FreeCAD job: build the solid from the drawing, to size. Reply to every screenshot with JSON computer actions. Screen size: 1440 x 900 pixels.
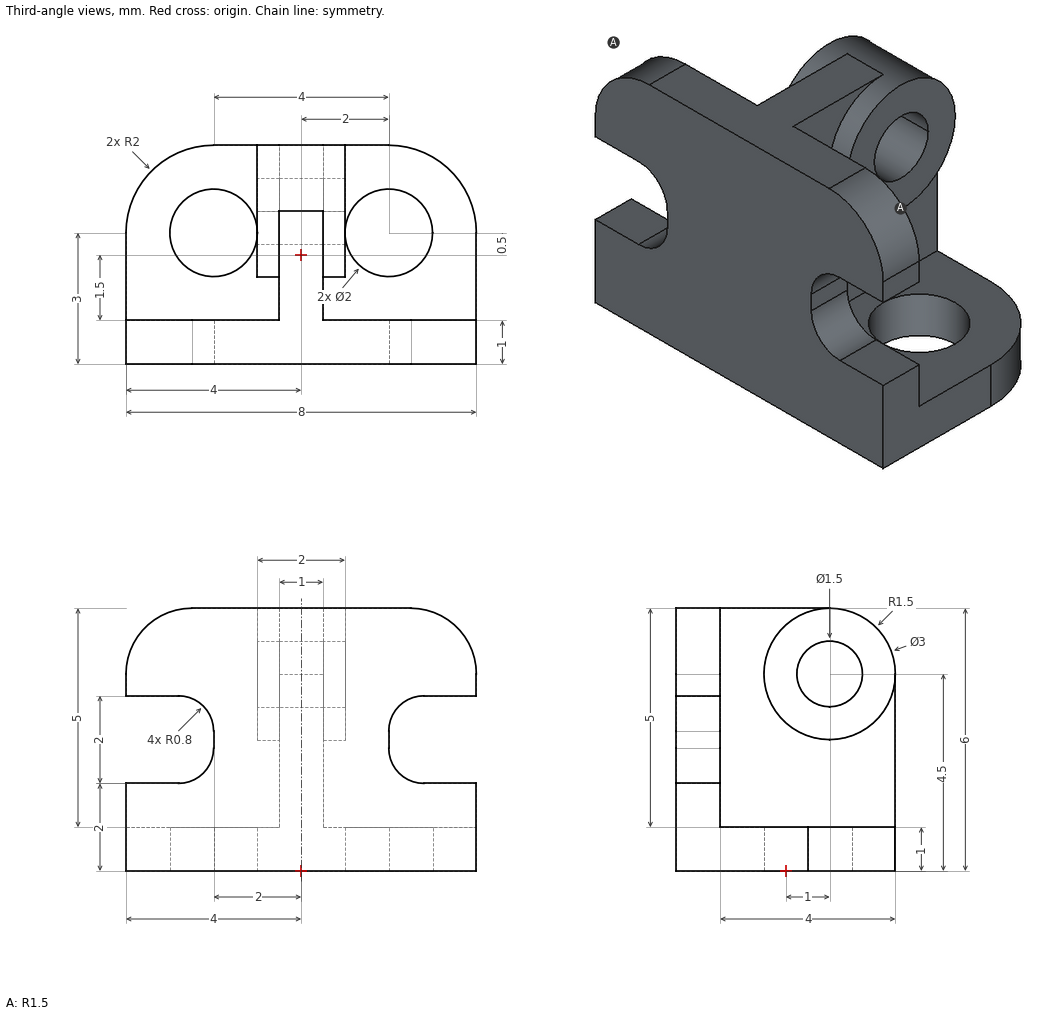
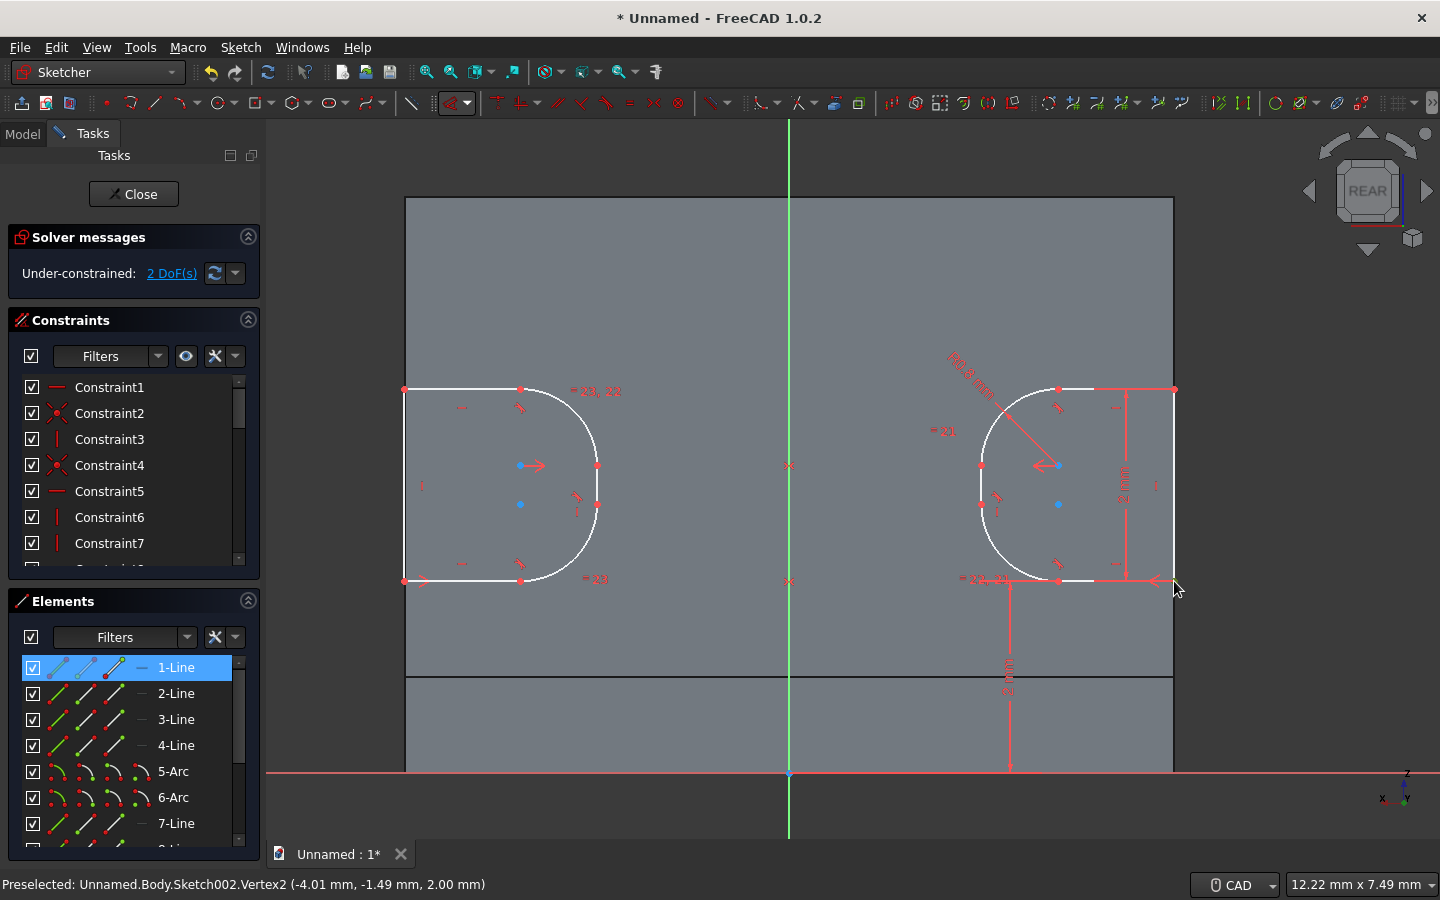
{"action": "left_click", "coordinate": [470, 104]}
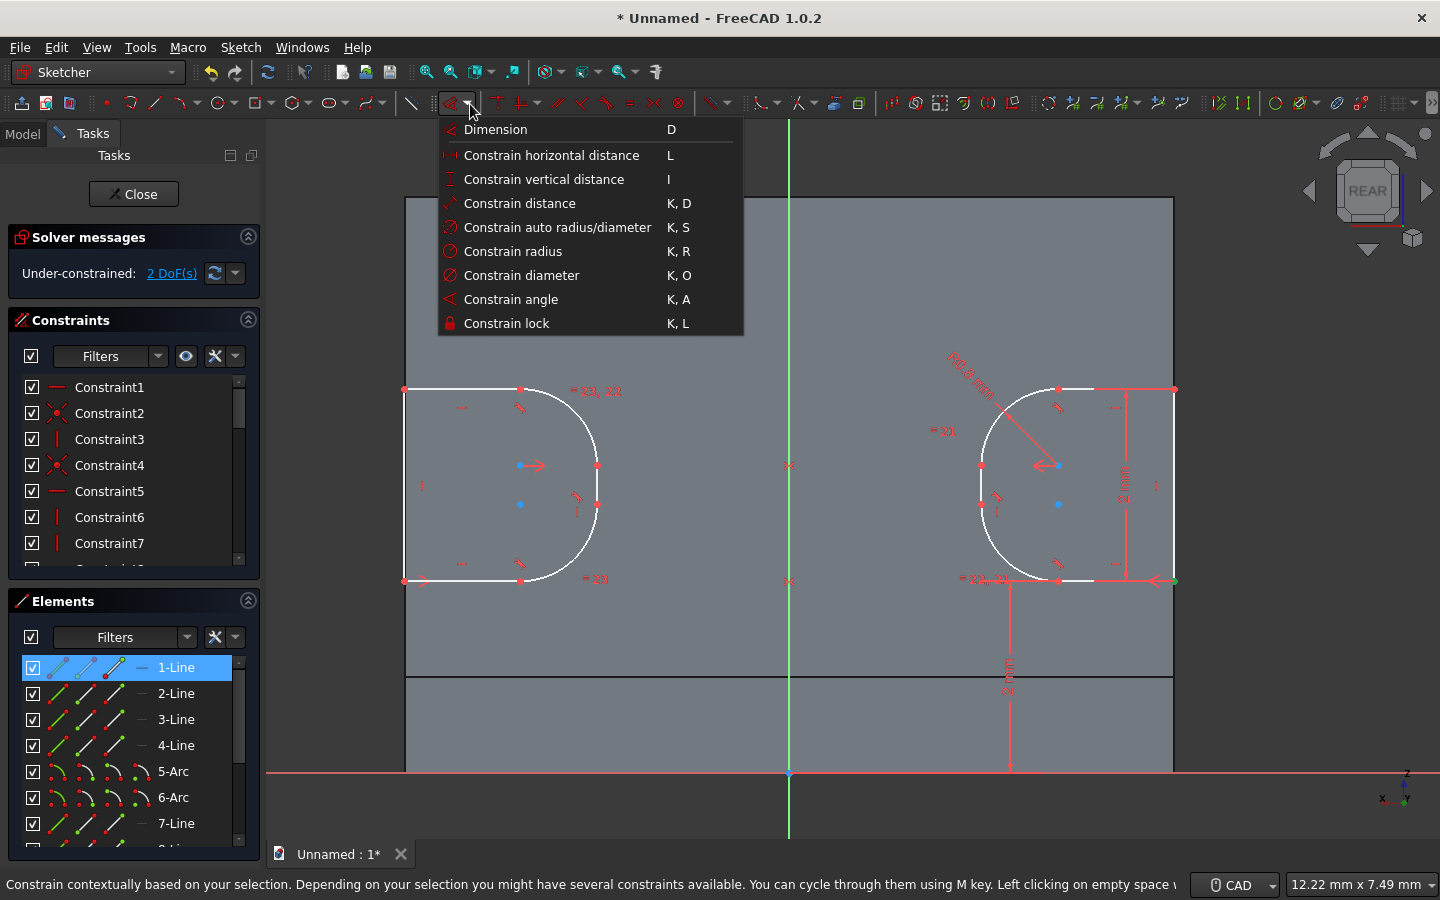
{"action": "left_click", "coordinate": [591, 155]}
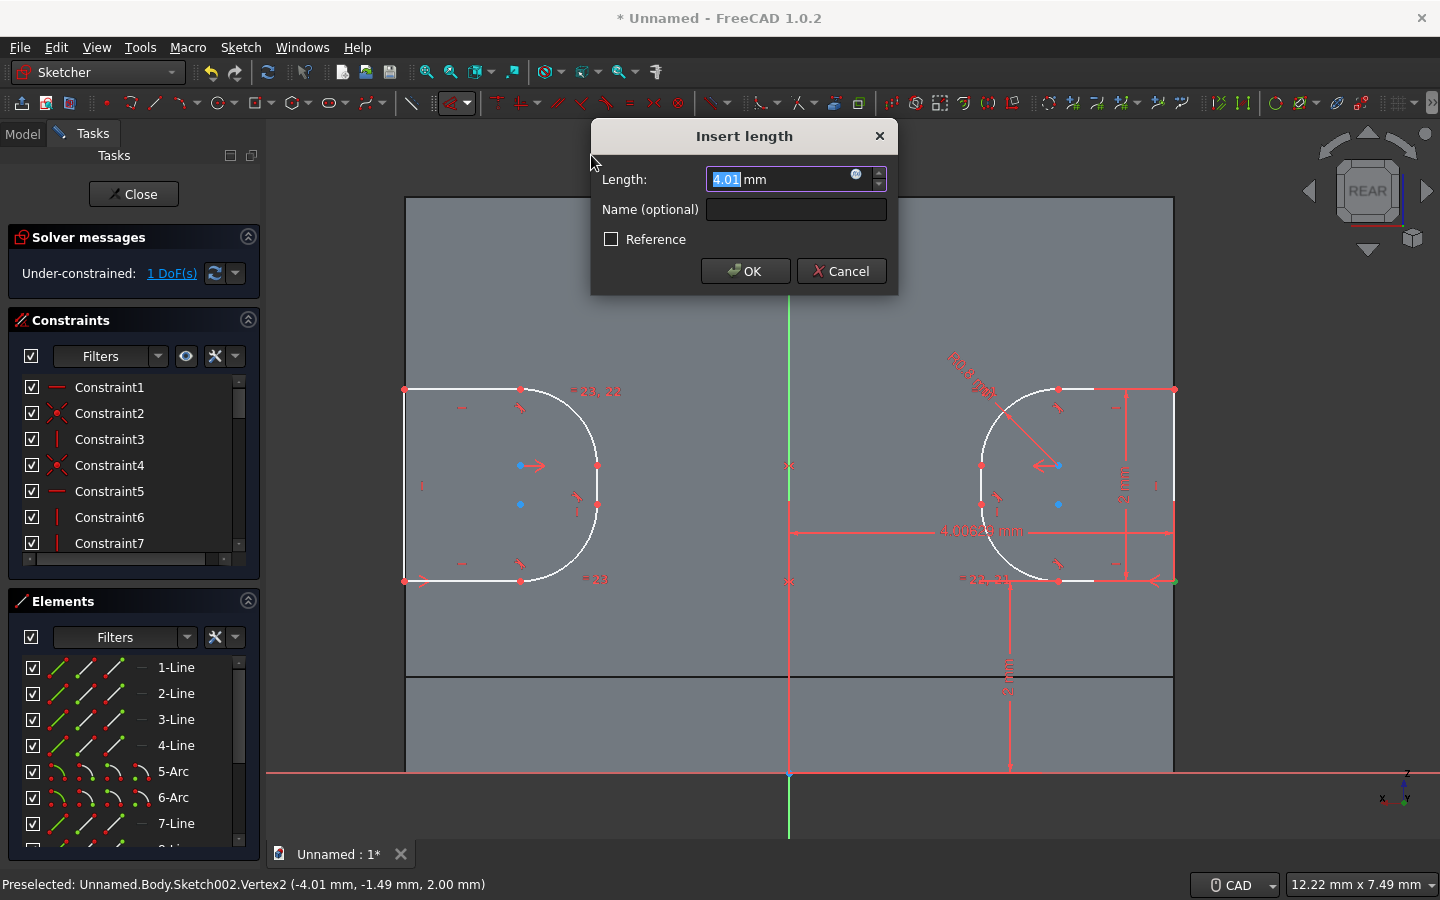
{"action": "type", "text": "4"}
{"action": "key", "text": "Return"}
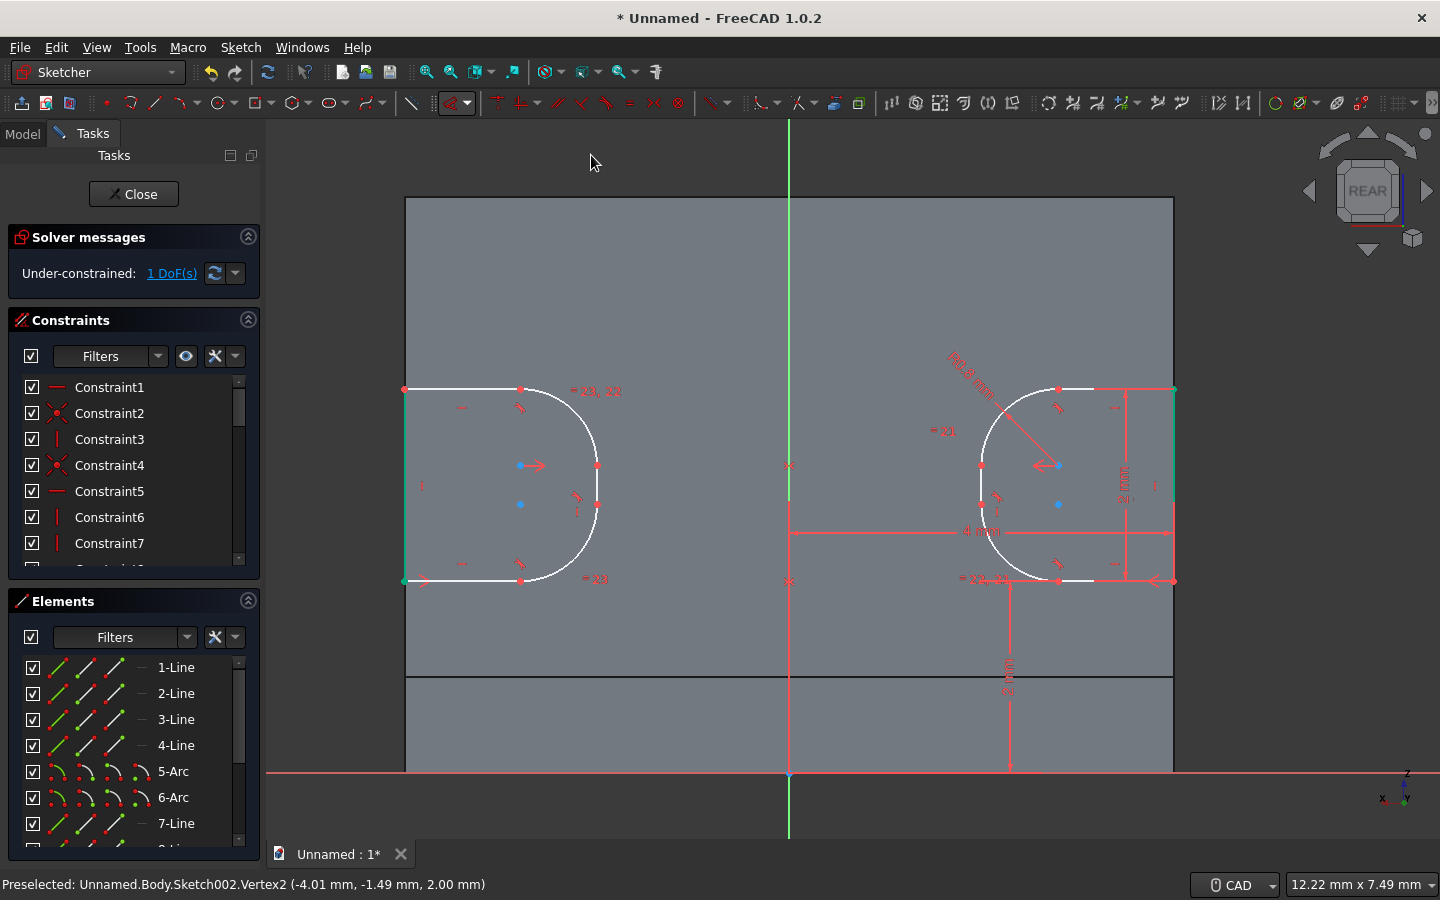
{"action": "left_click", "coordinate": [981, 466]}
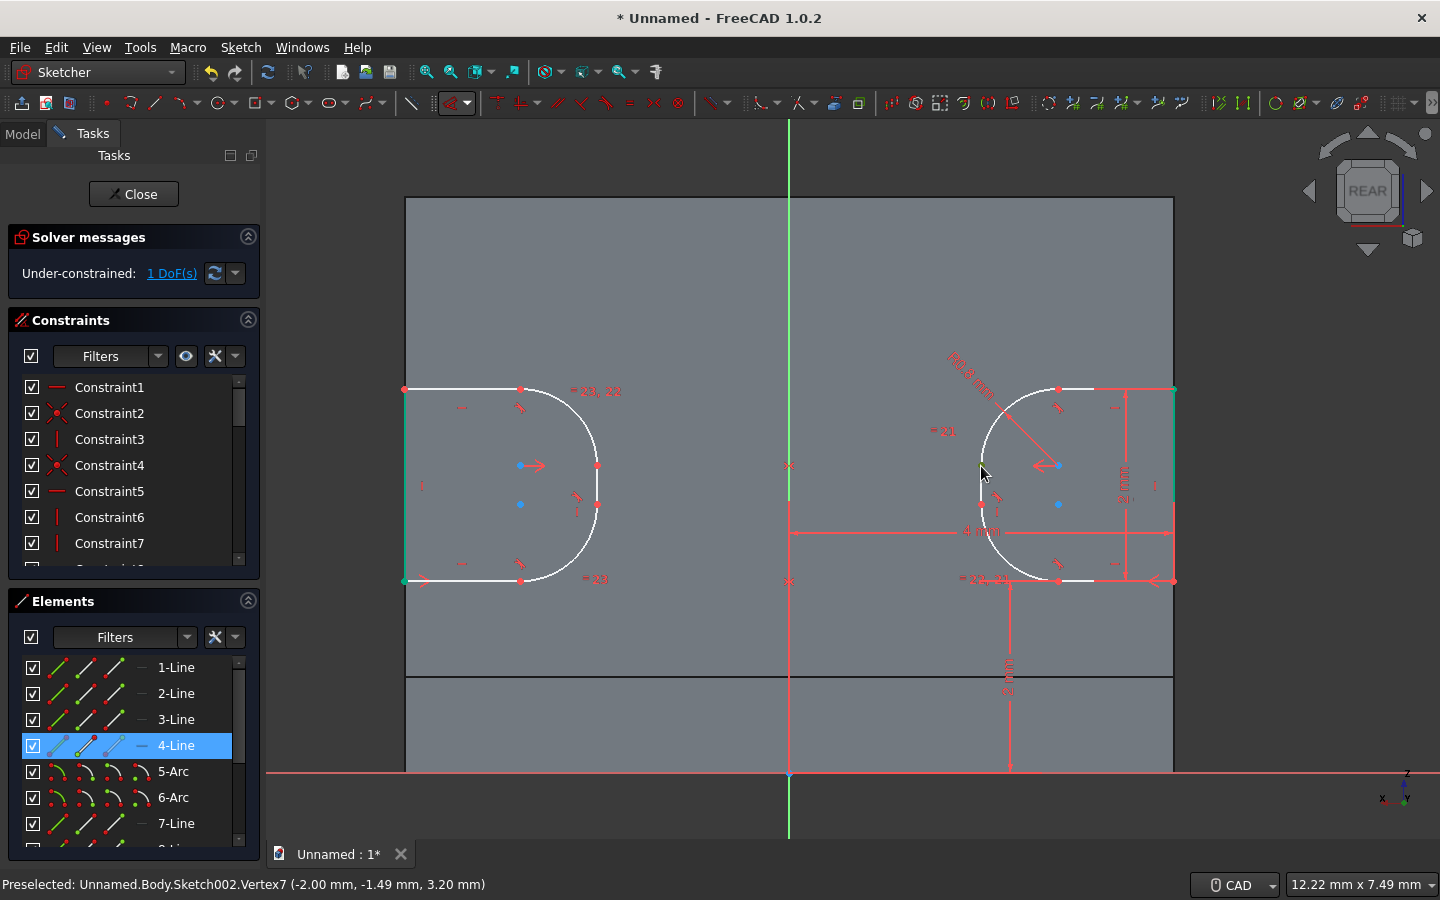
{"action": "left_click", "coordinate": [470, 104]}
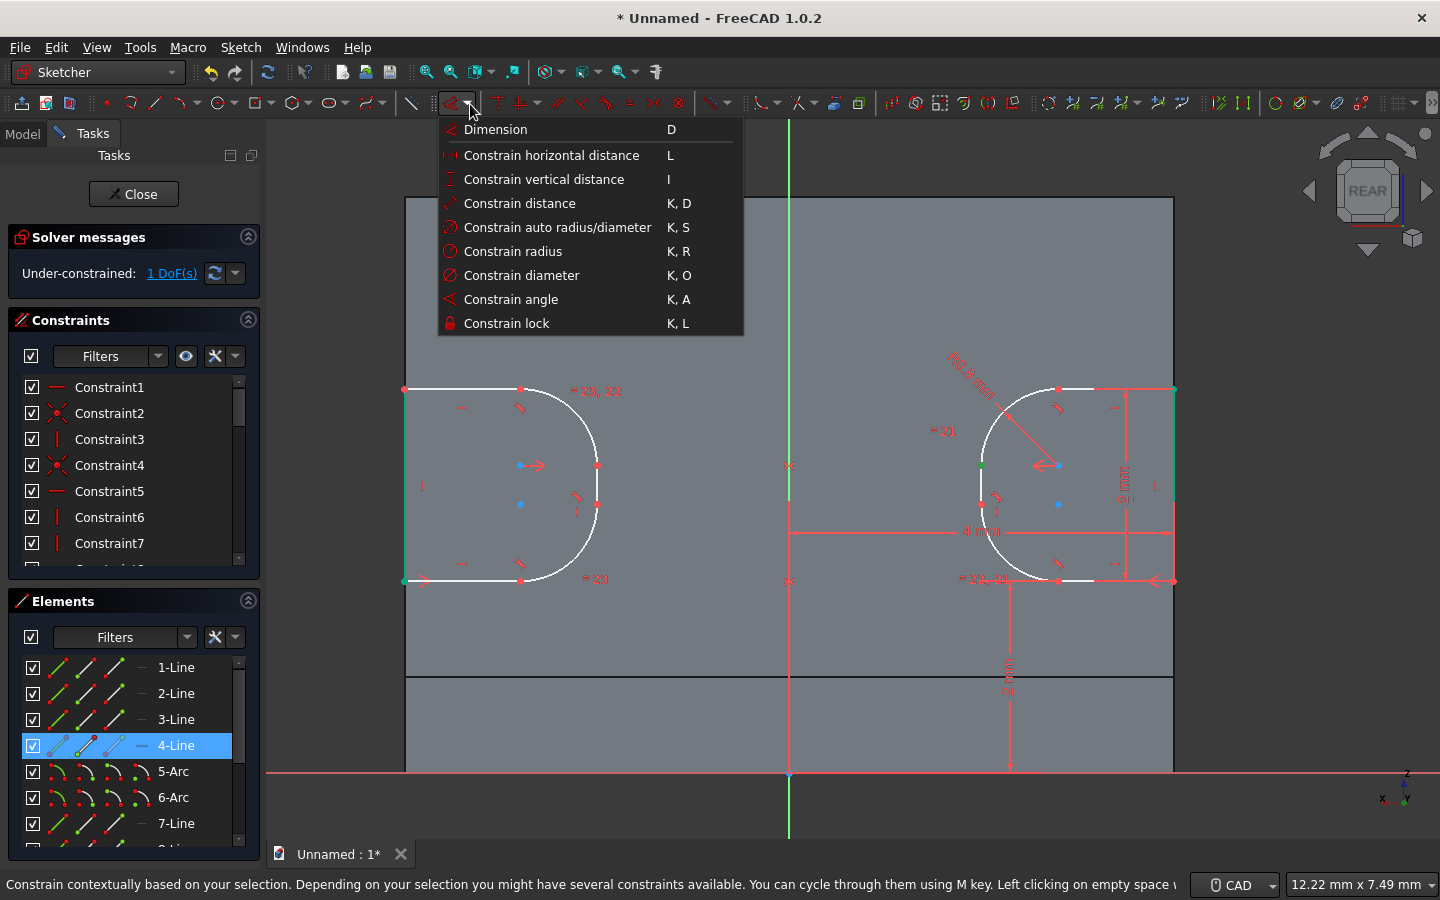
{"action": "left_click", "coordinate": [591, 155]}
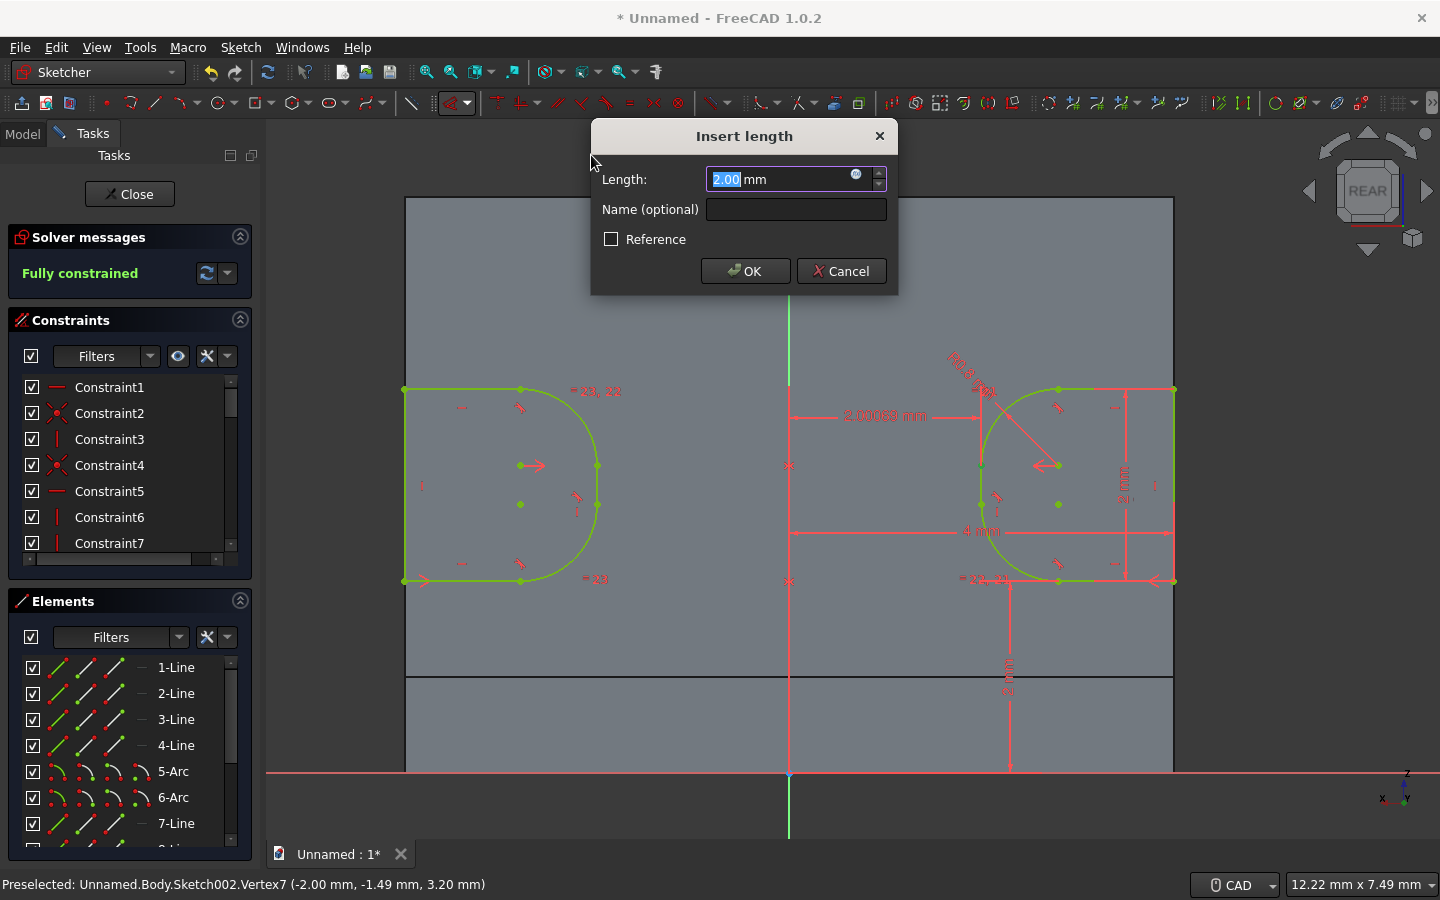
{"action": "type", "text": "2"}
{"action": "key", "text": "Return"}